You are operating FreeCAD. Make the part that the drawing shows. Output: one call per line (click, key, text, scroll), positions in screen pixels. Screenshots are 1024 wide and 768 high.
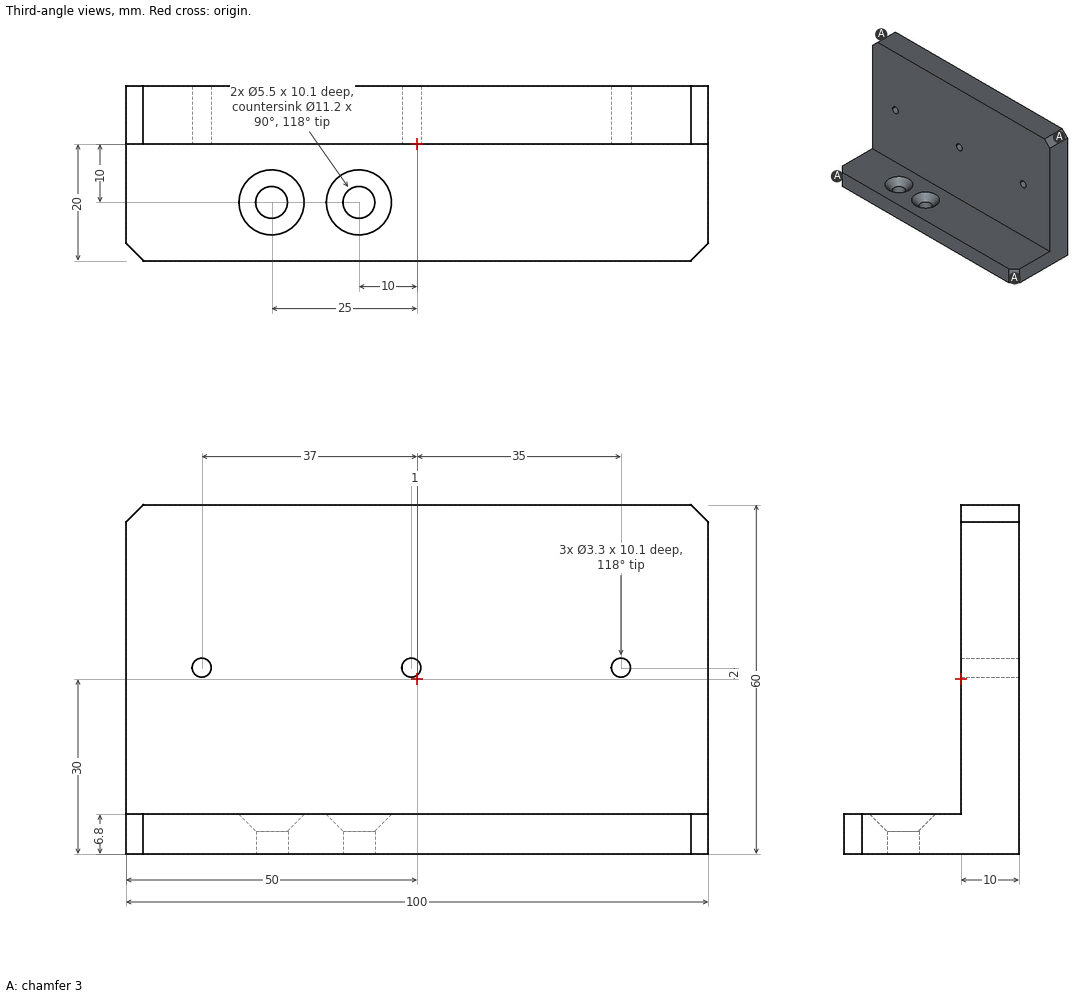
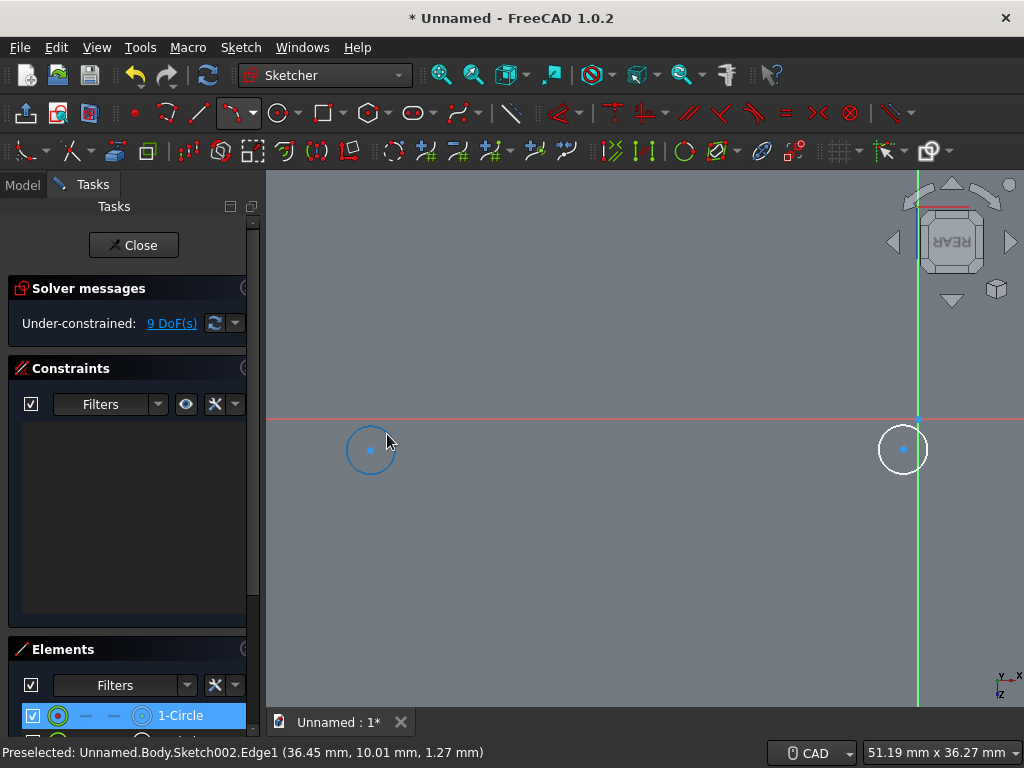
click(388, 433)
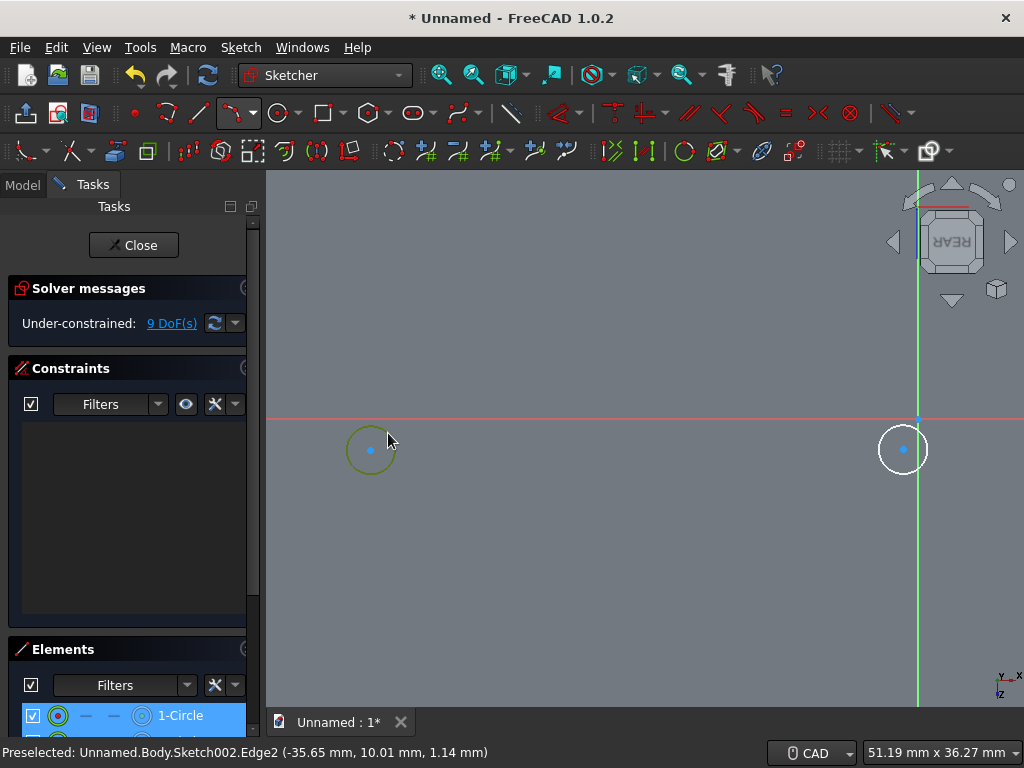
scroll(386, 434, down, 5)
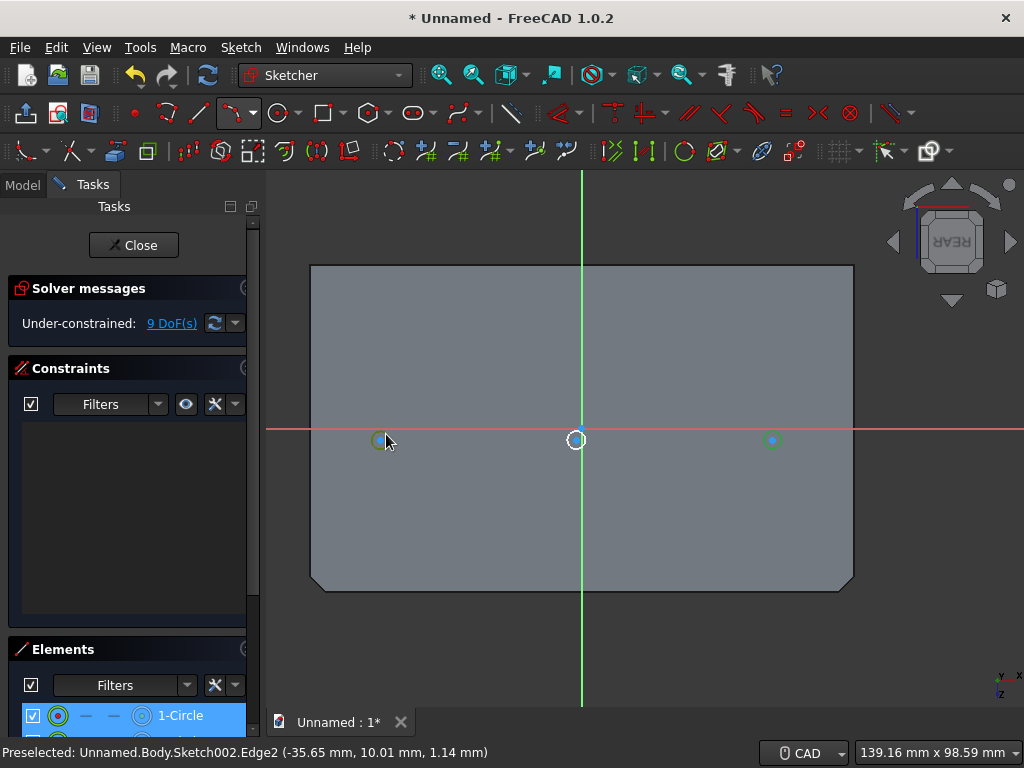
scroll(583, 434, up, 6)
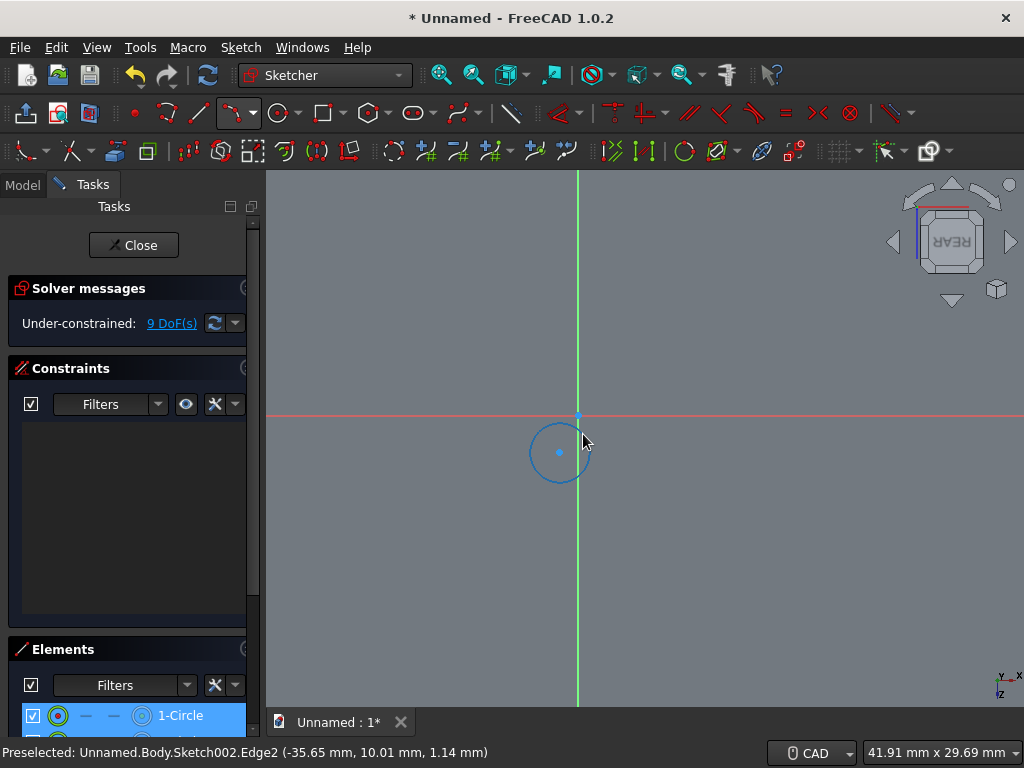
click(581, 432)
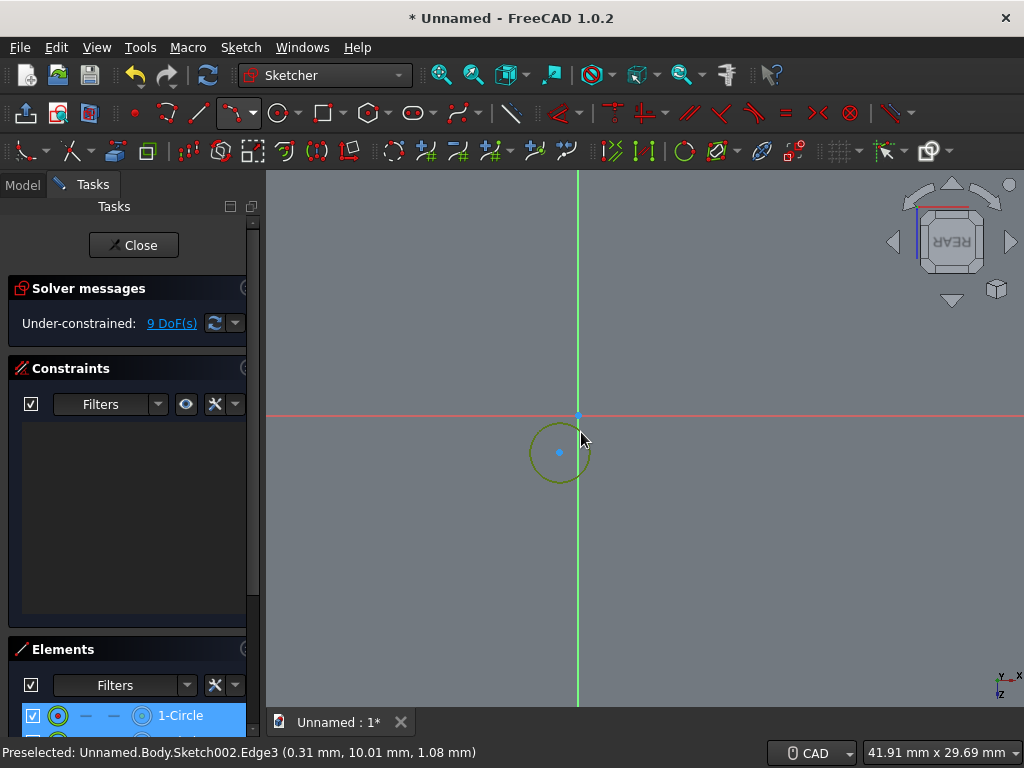
key(e)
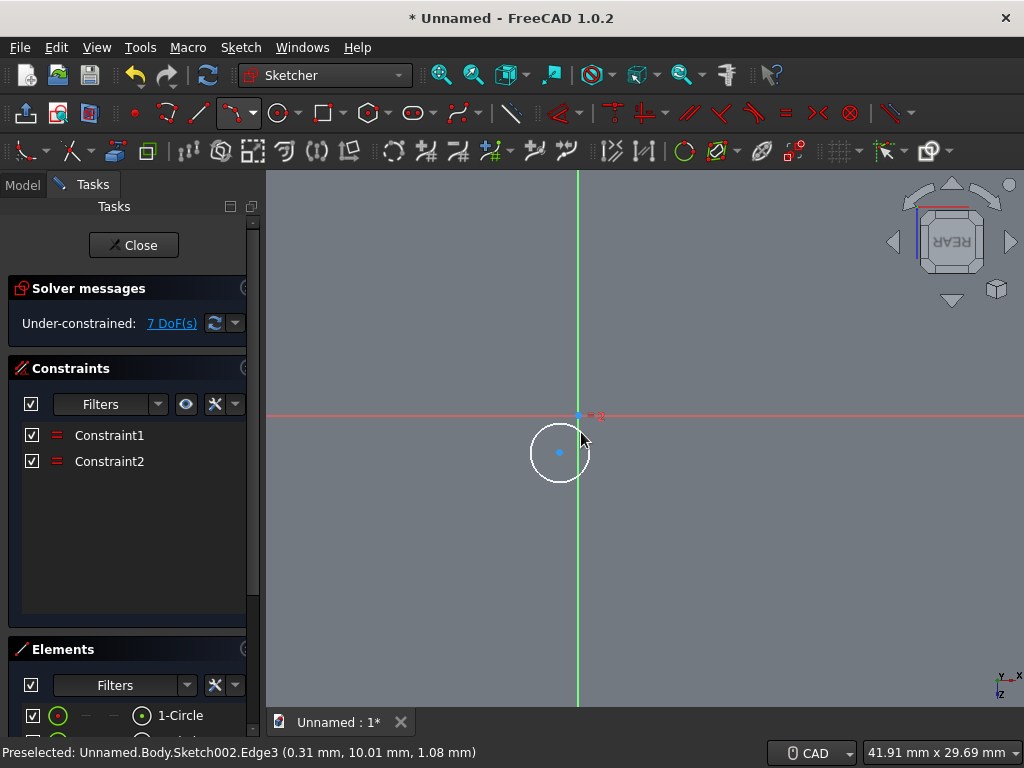
scroll(584, 434, down, 6)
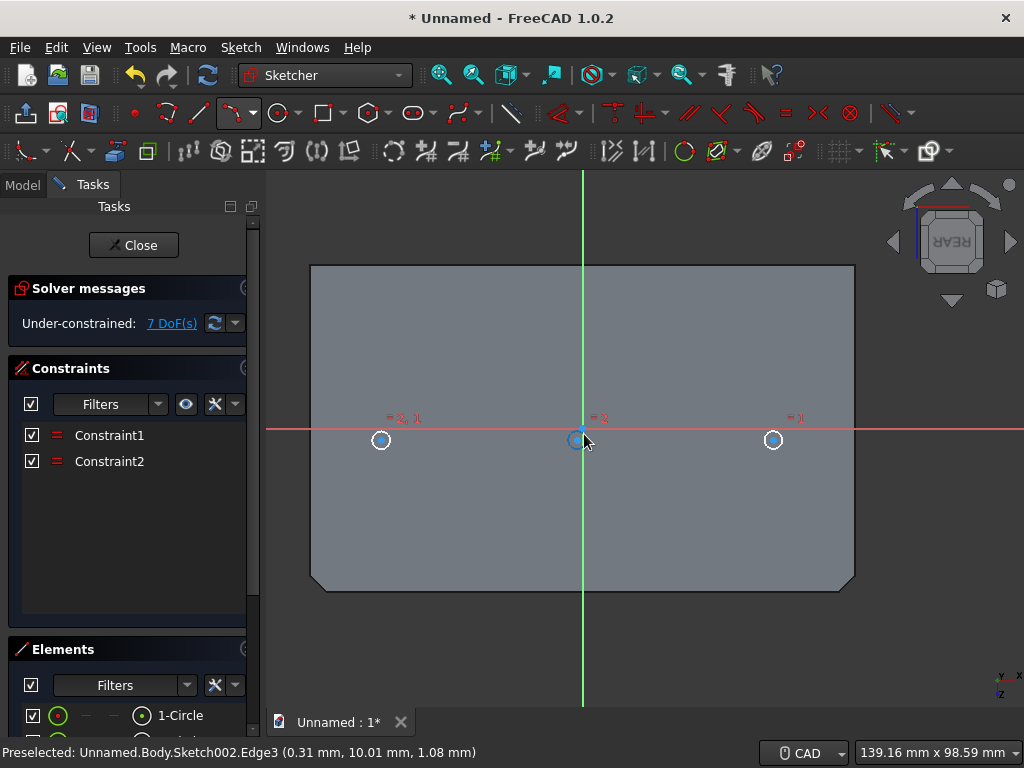
click(773, 440)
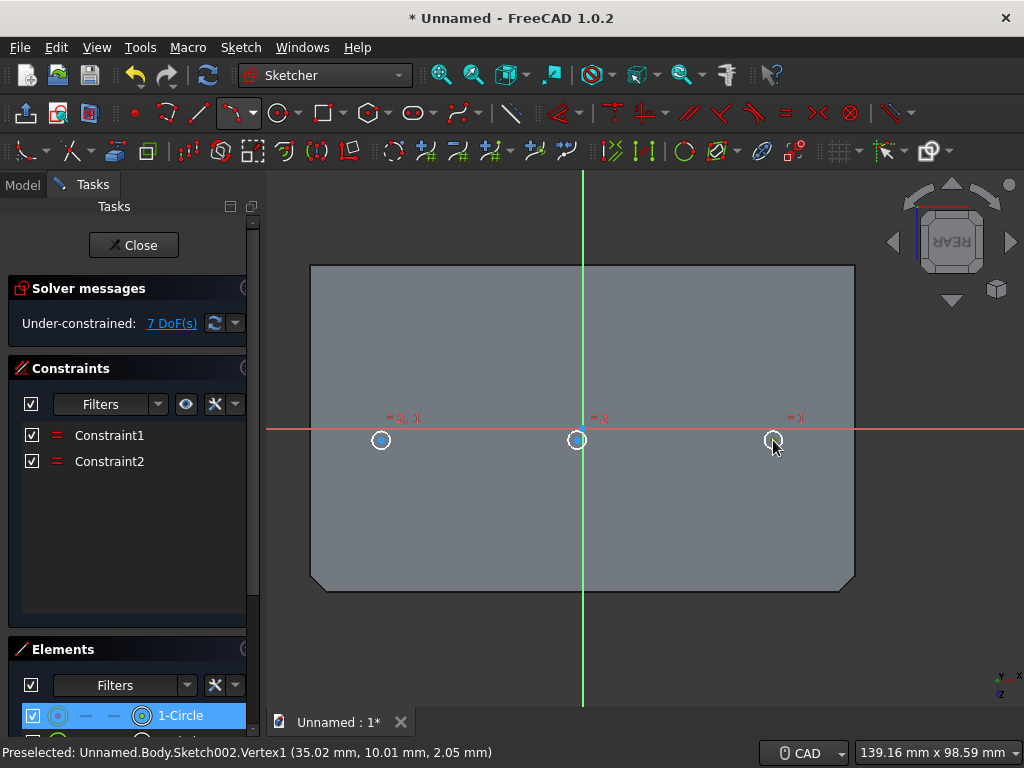
click(381, 440)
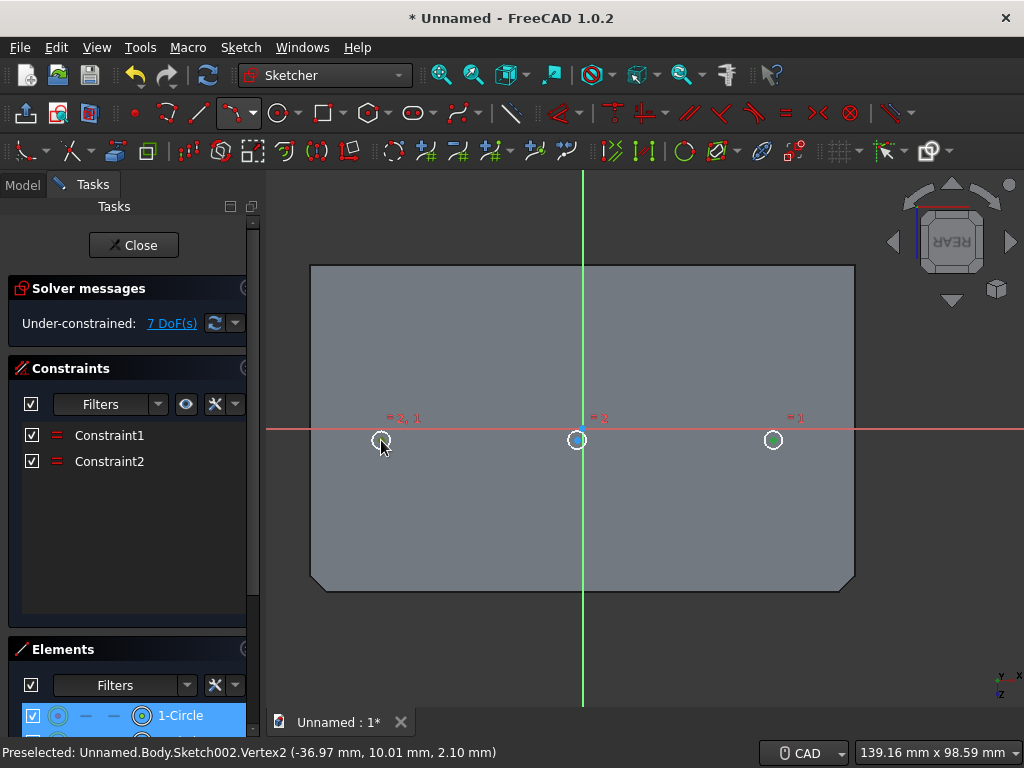
key(h)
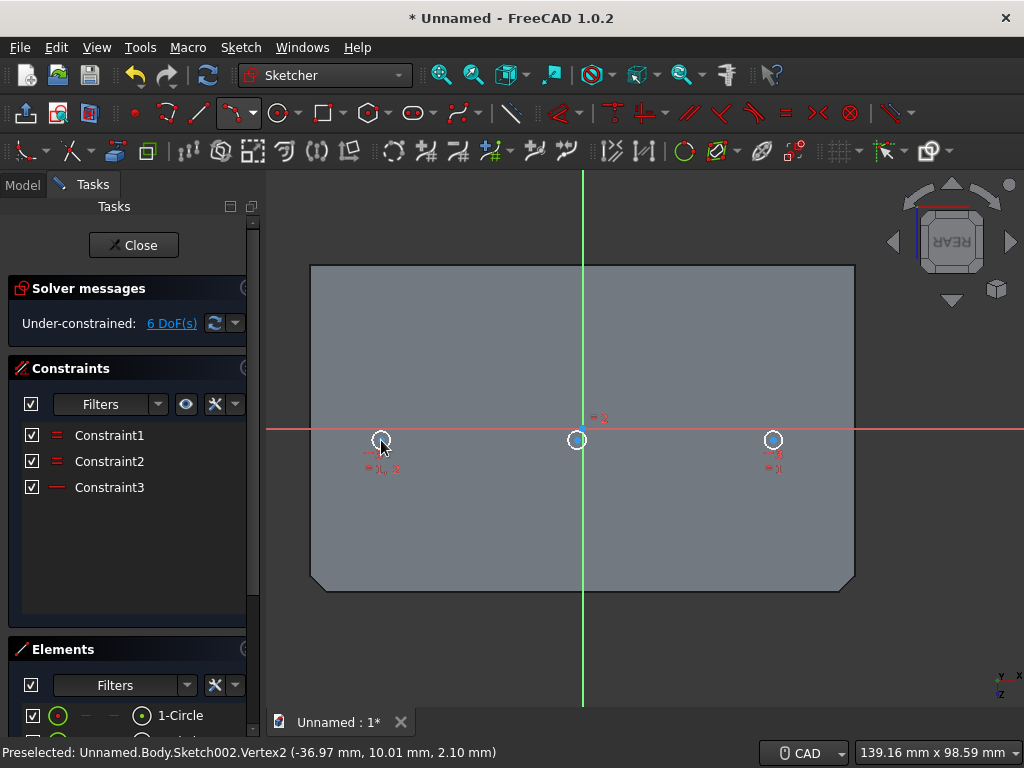
click(773, 440)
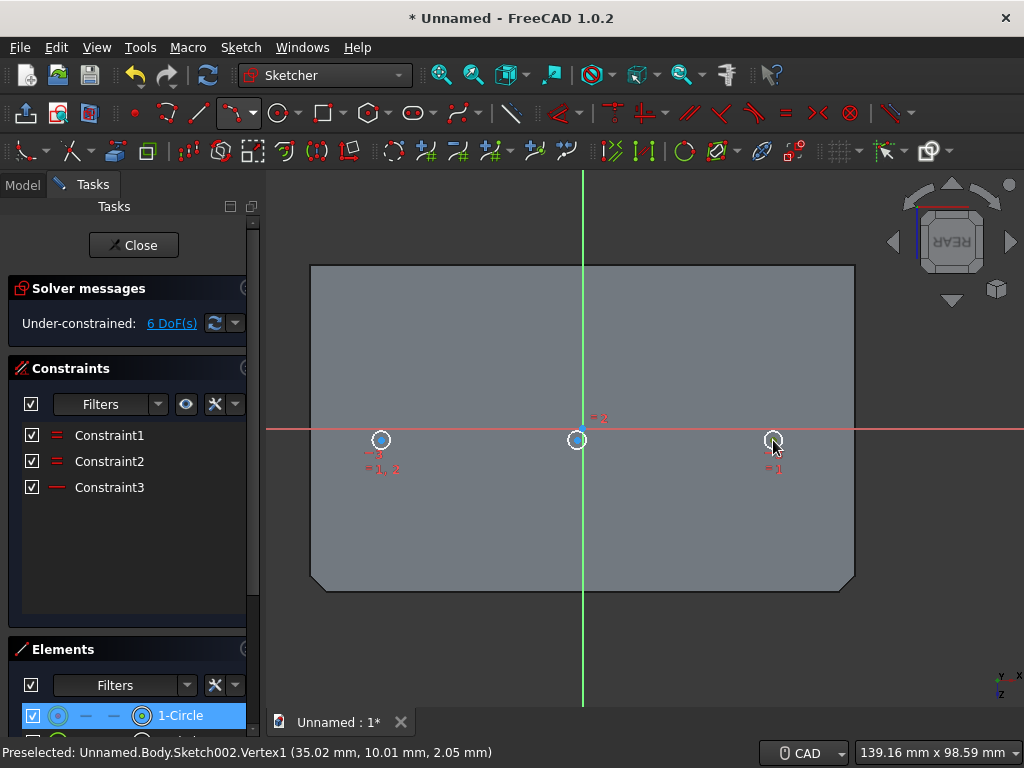
click(577, 440)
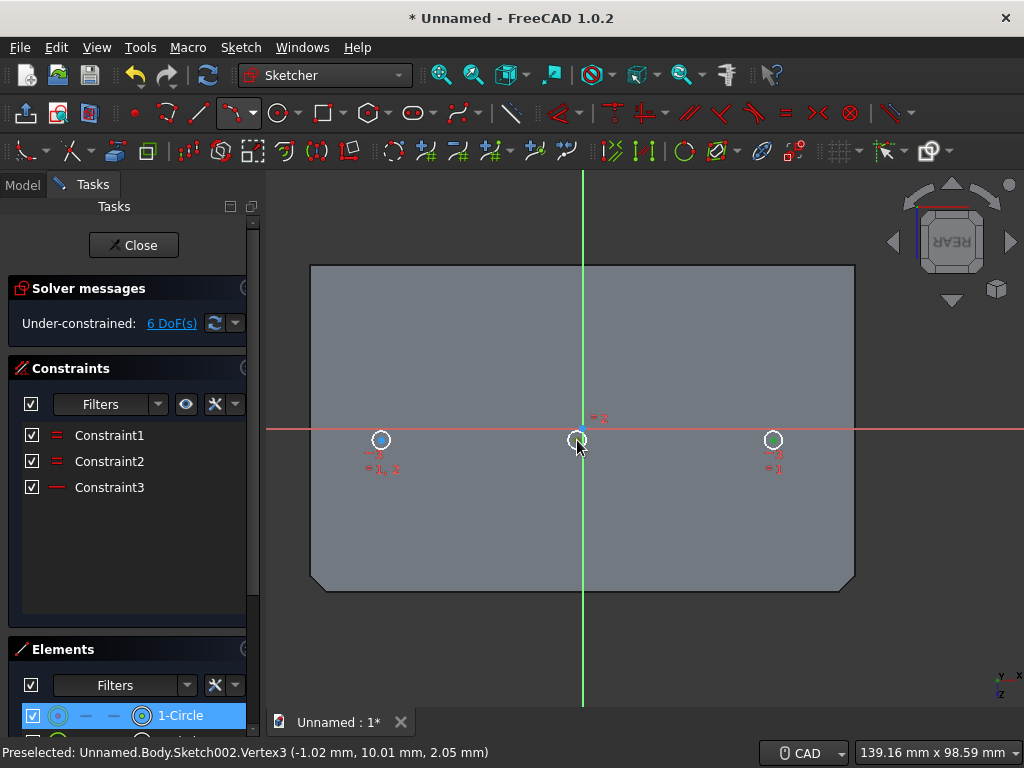
key(h)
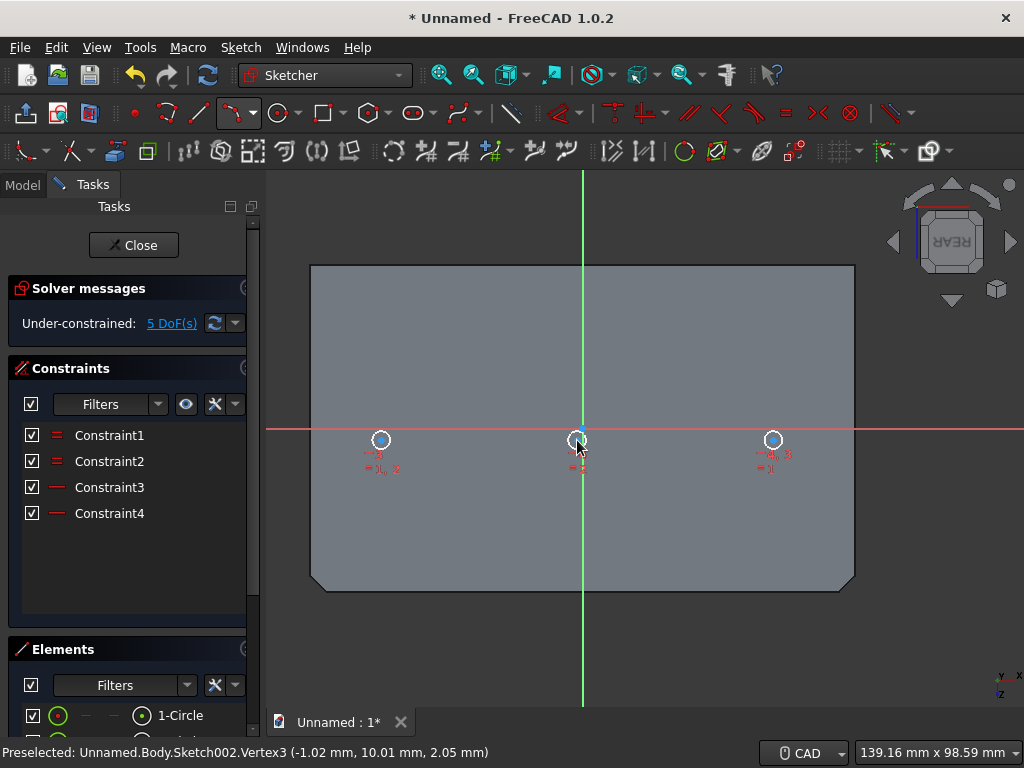
key(d)